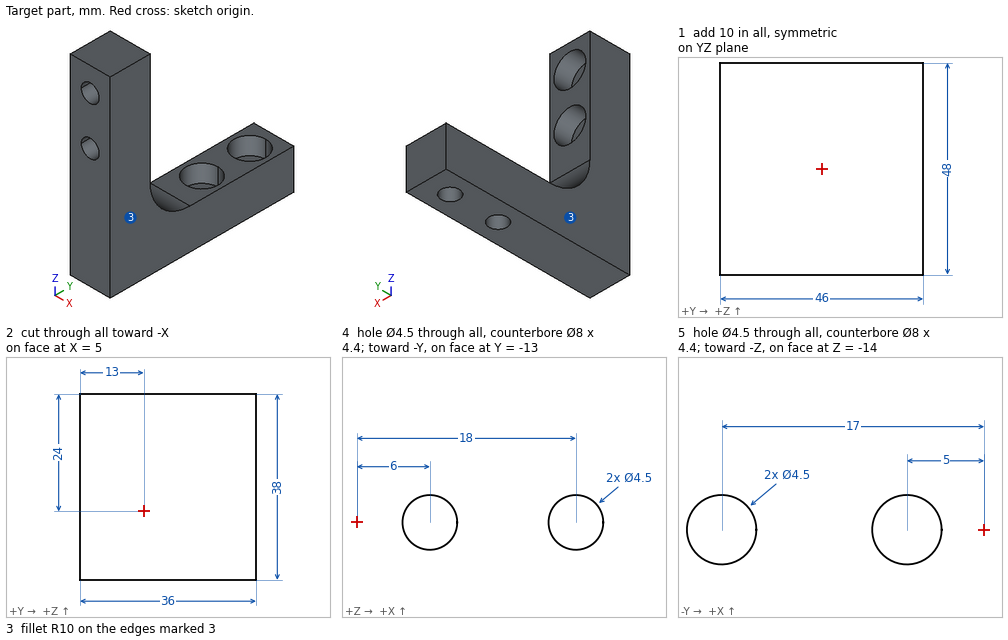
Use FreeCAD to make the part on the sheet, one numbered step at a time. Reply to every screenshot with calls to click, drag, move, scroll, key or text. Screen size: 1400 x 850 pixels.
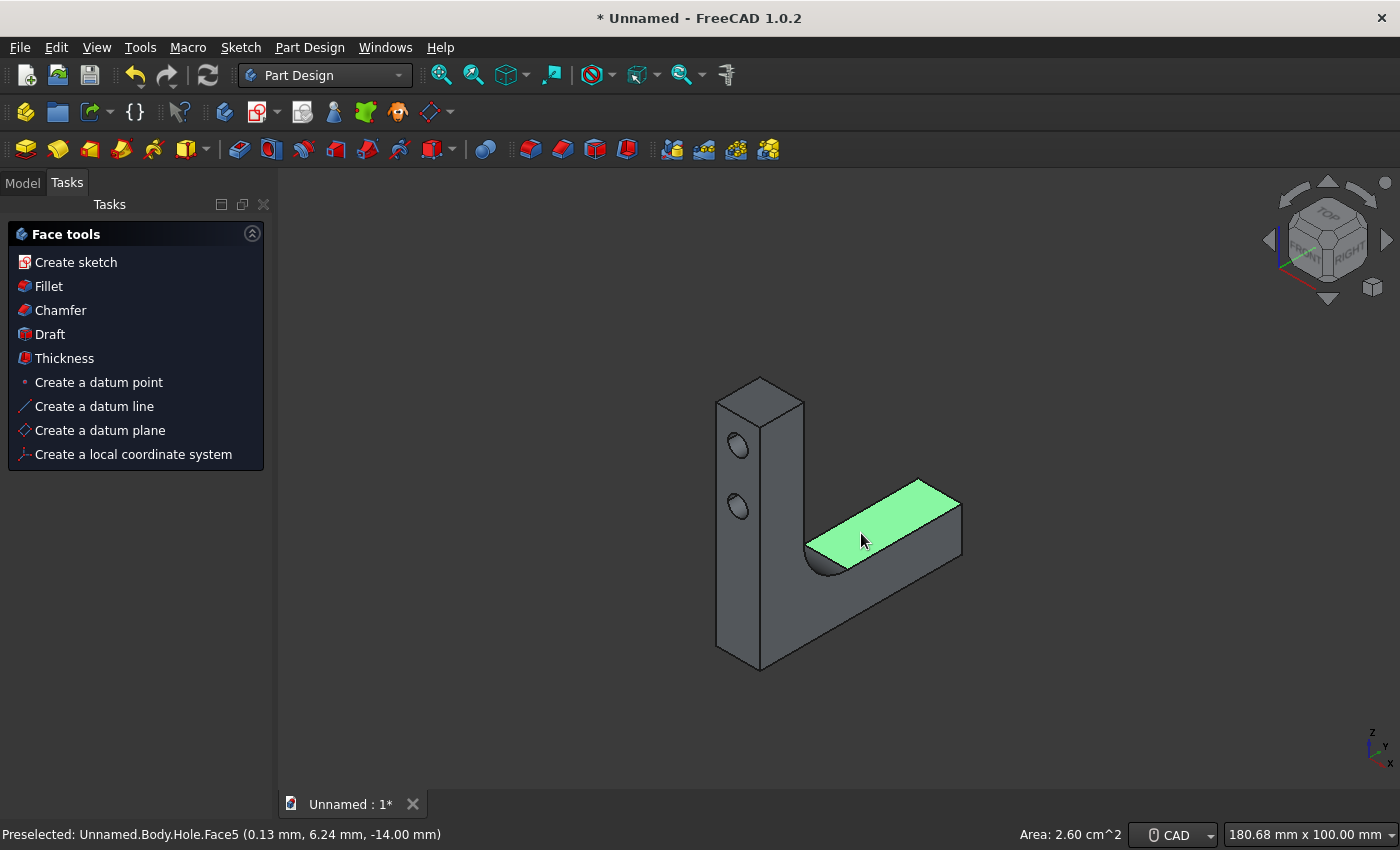
click(258, 112)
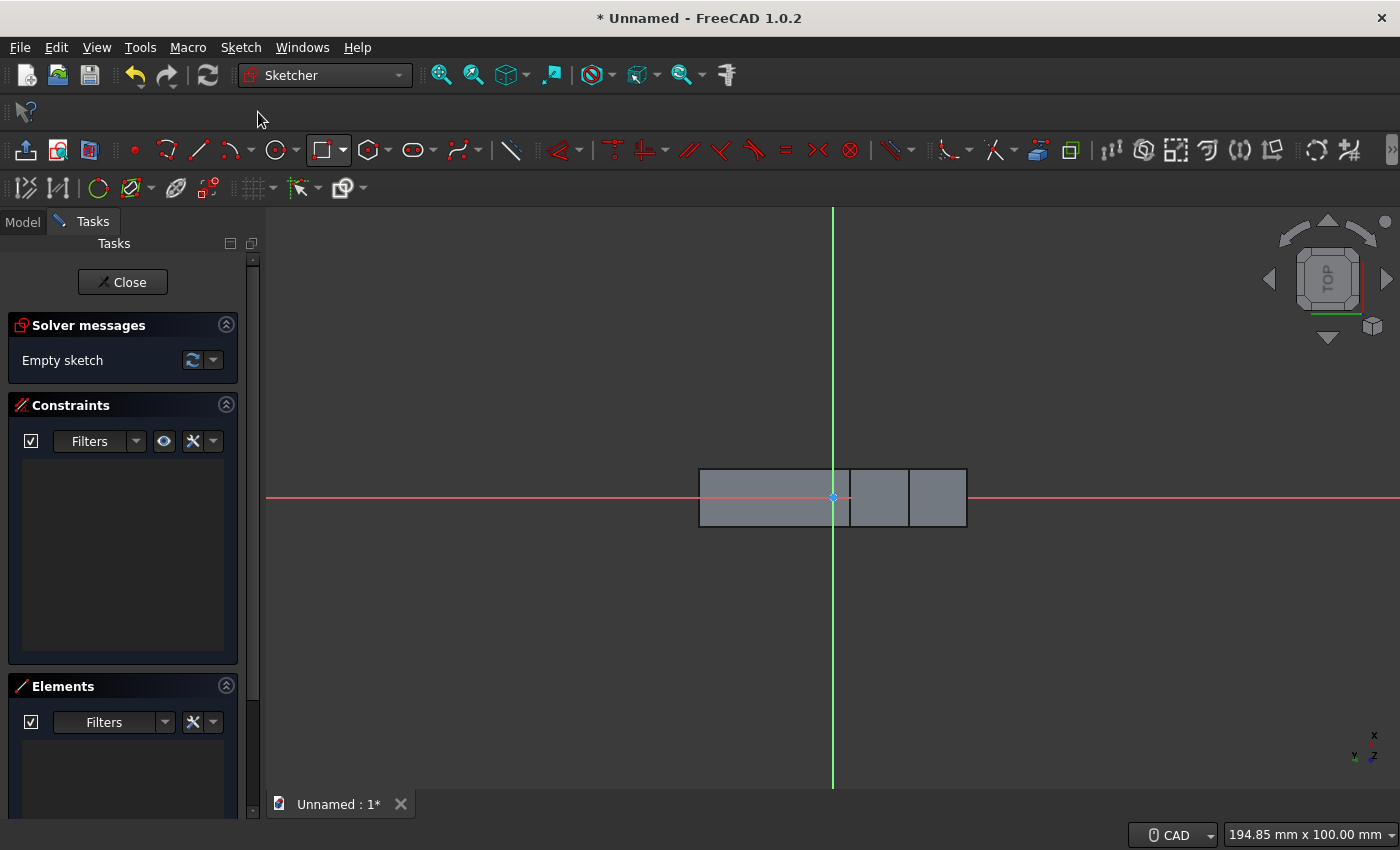
click(90, 150)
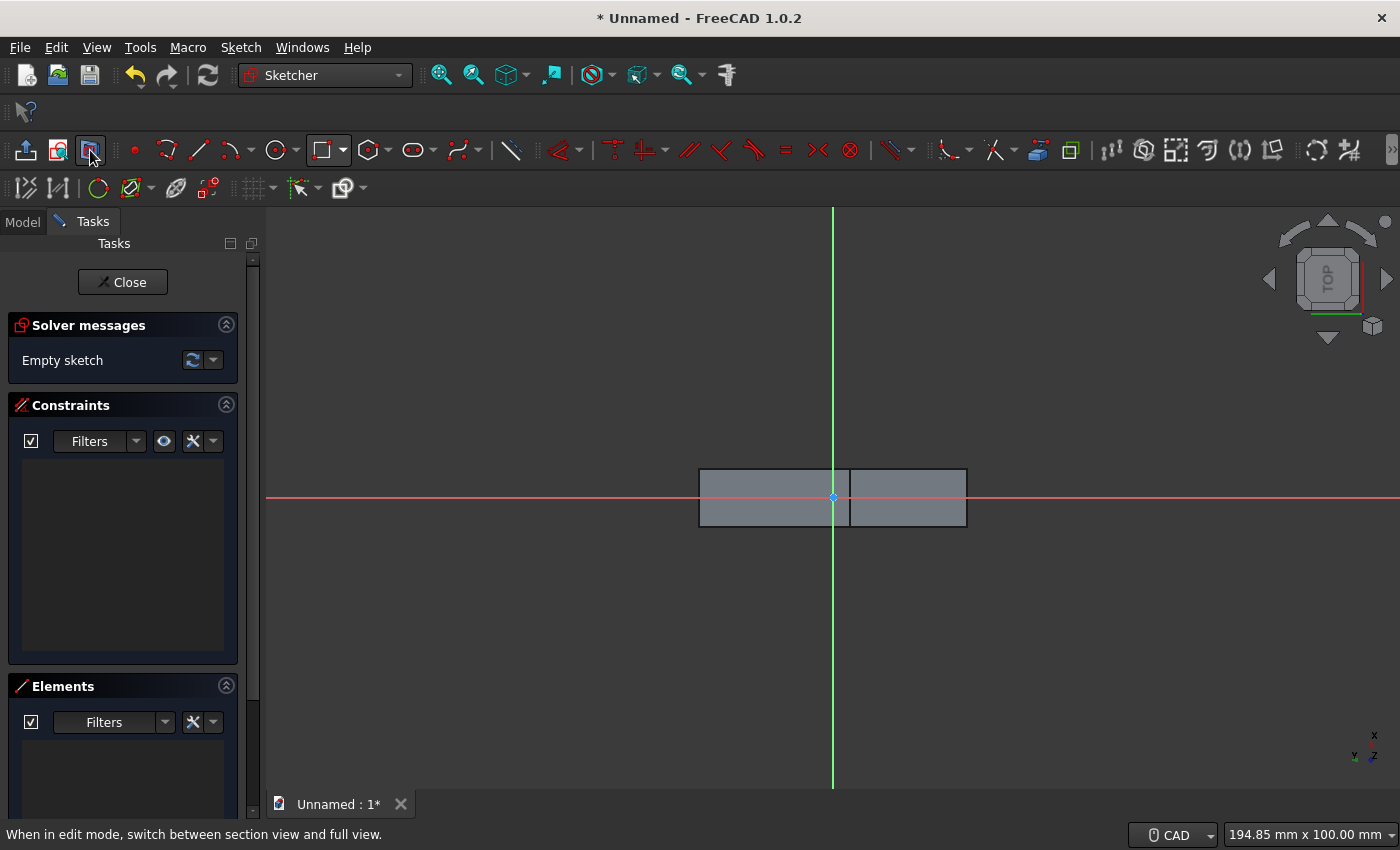
scroll(779, 498, up, 9)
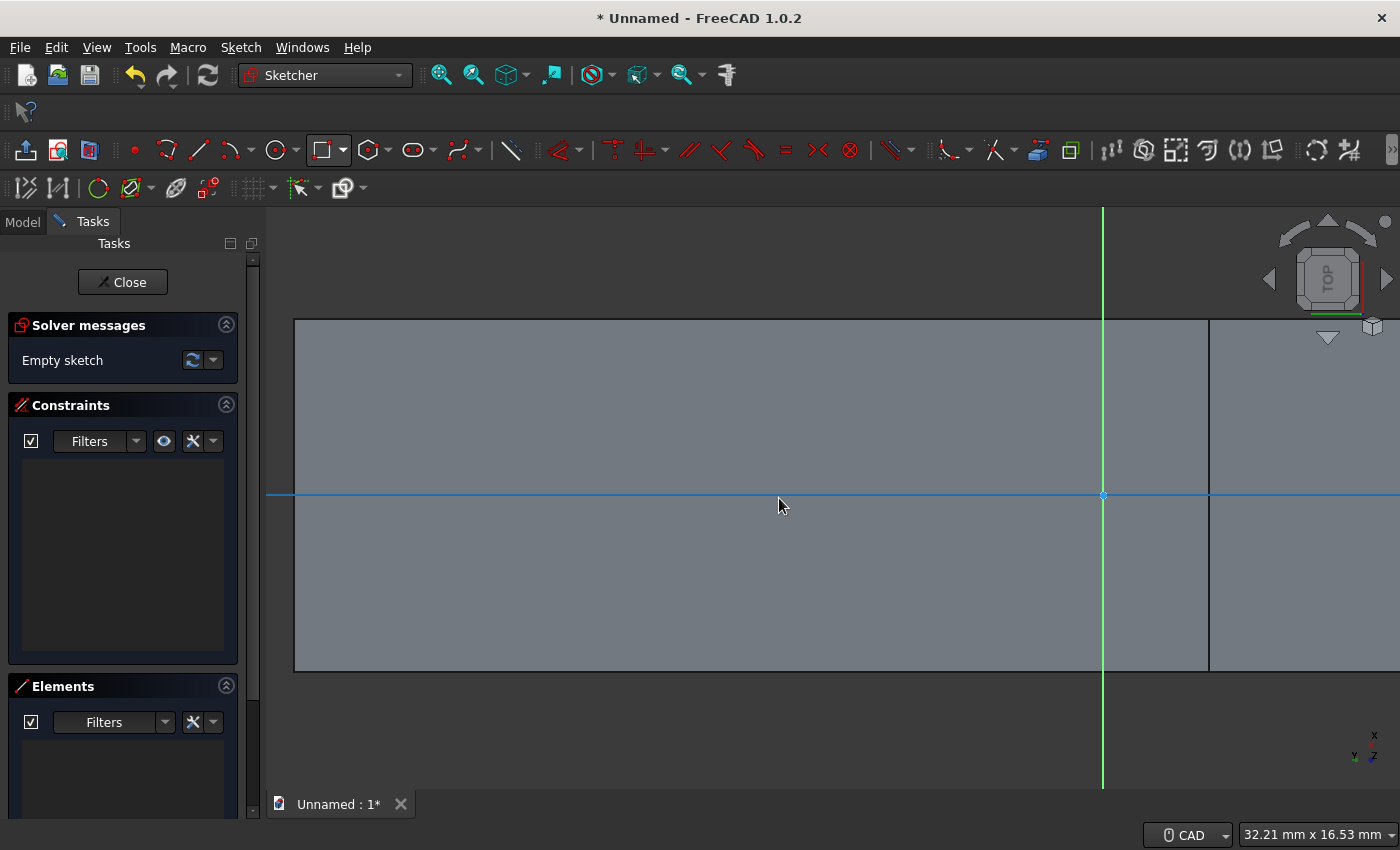
click(276, 150)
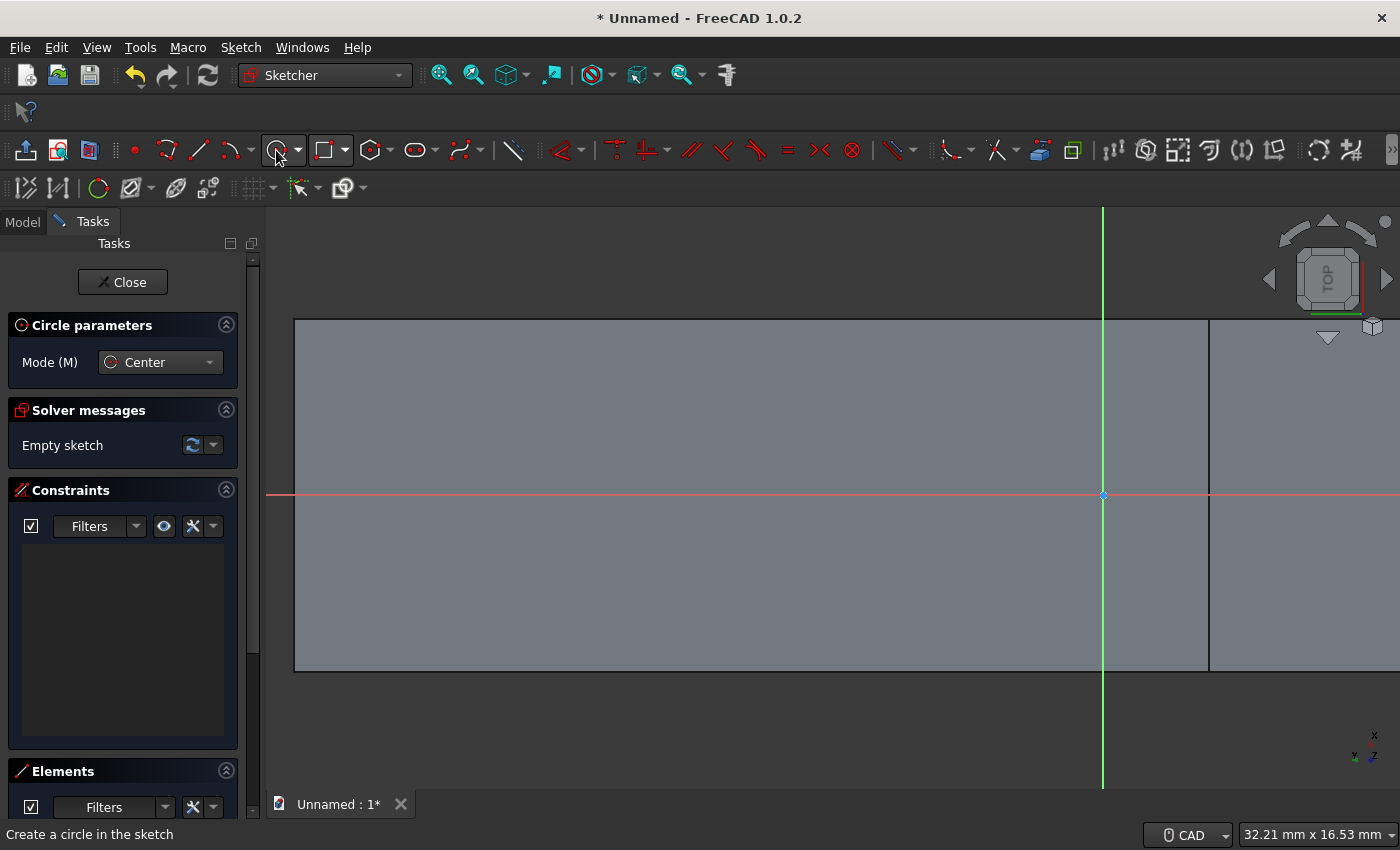
click(505, 495)
move(561, 439)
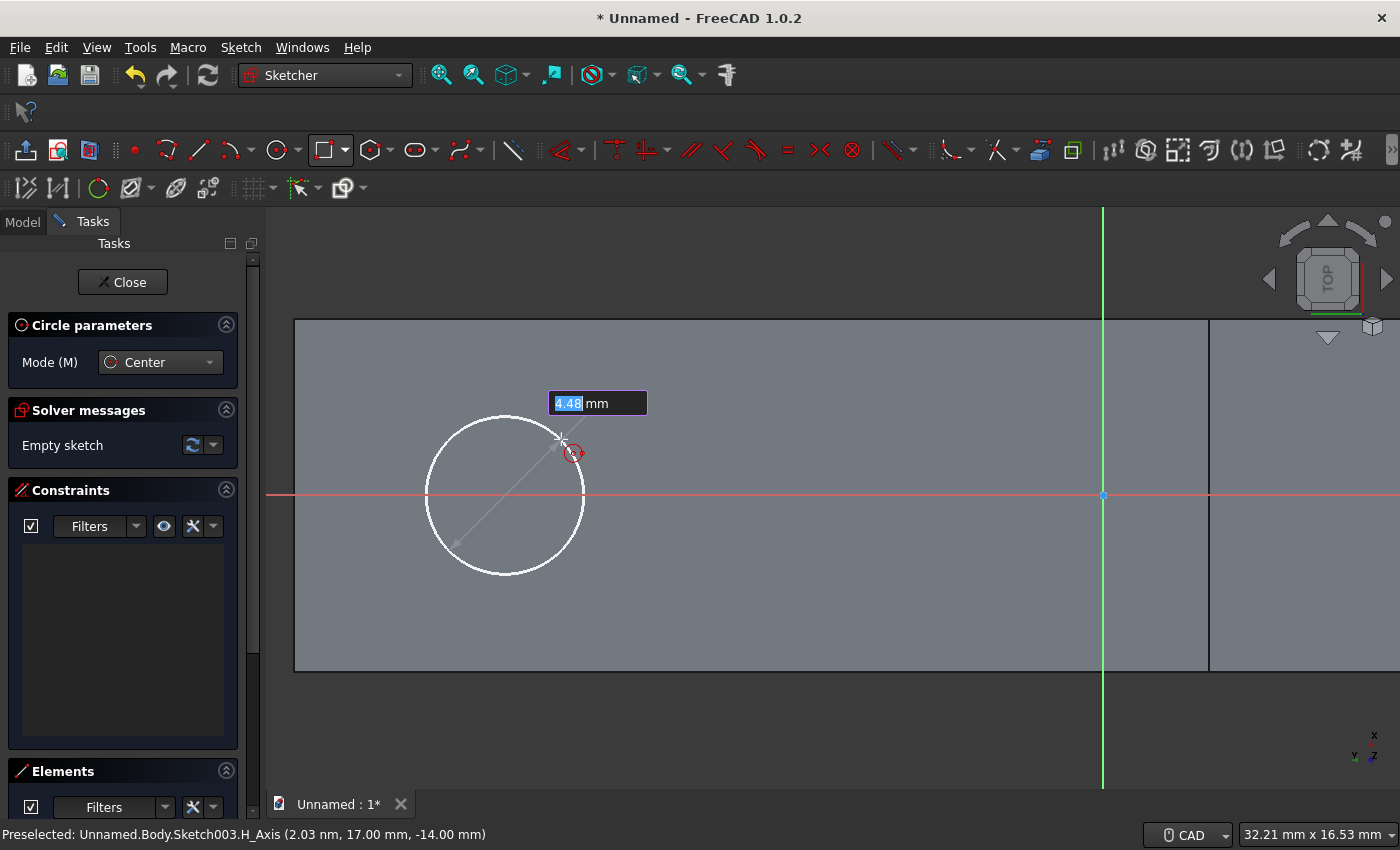
text(4.5)
key(Return)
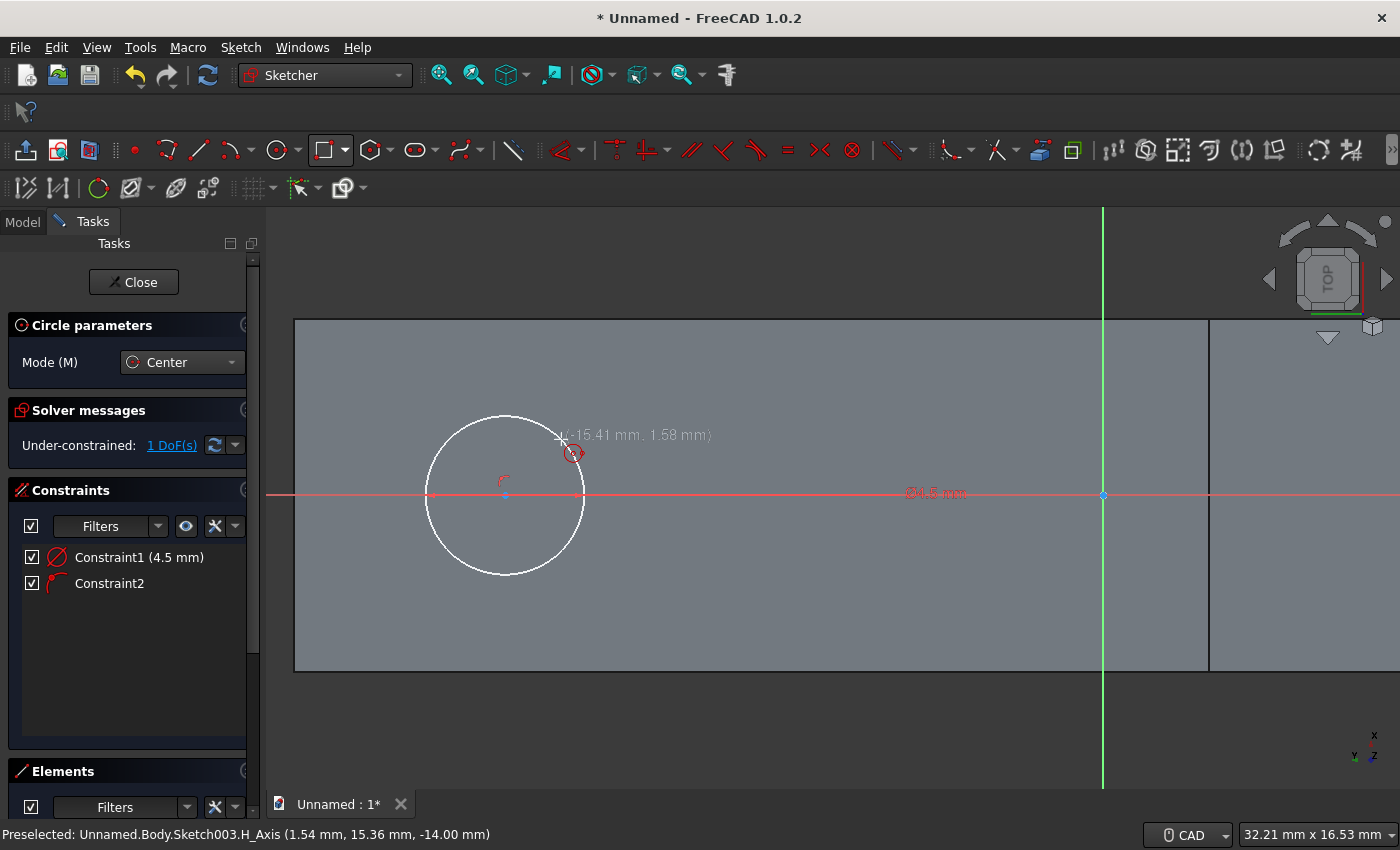
click(927, 495)
move(983, 439)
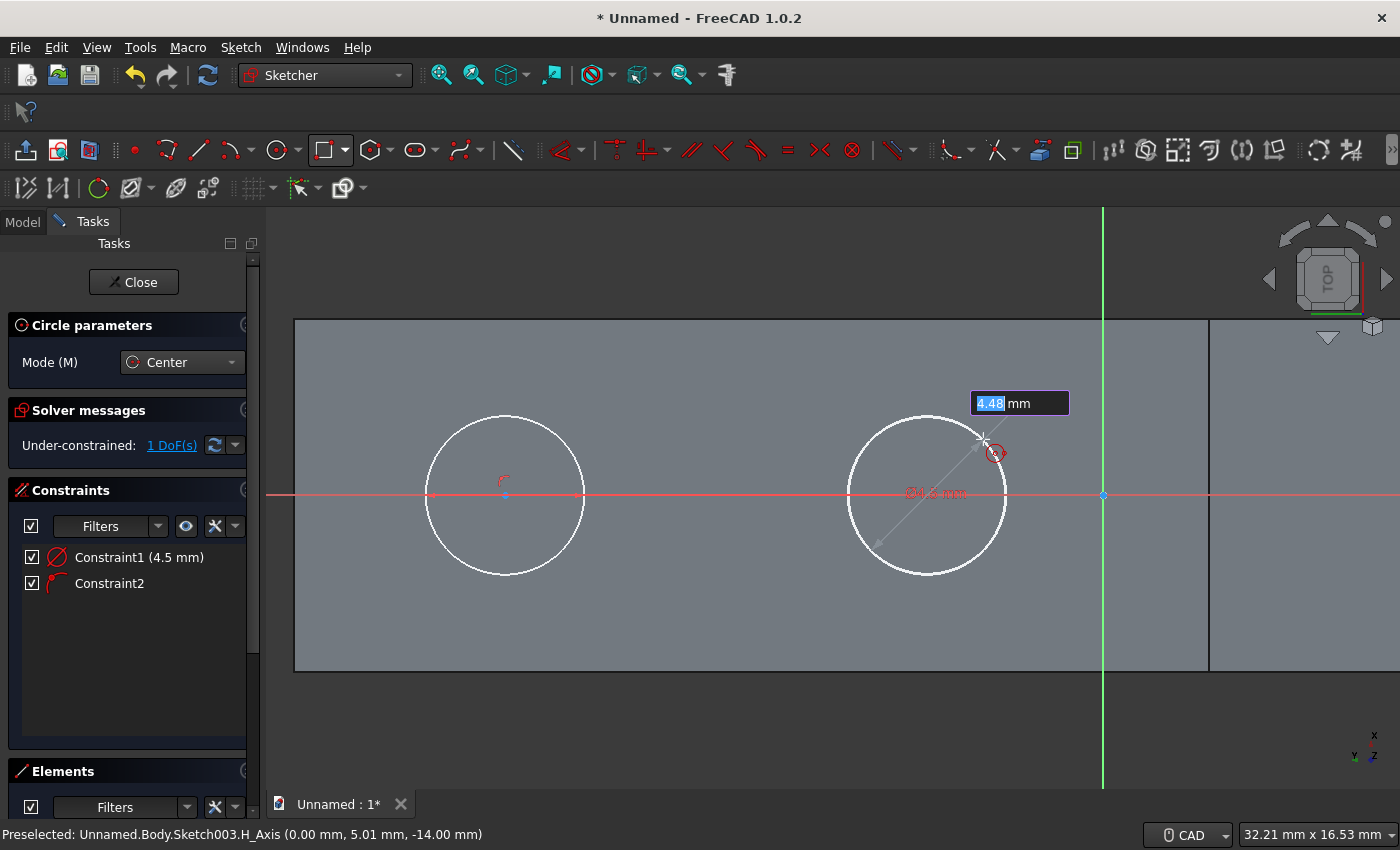
text(4.5)
key(Return)
key(Escape)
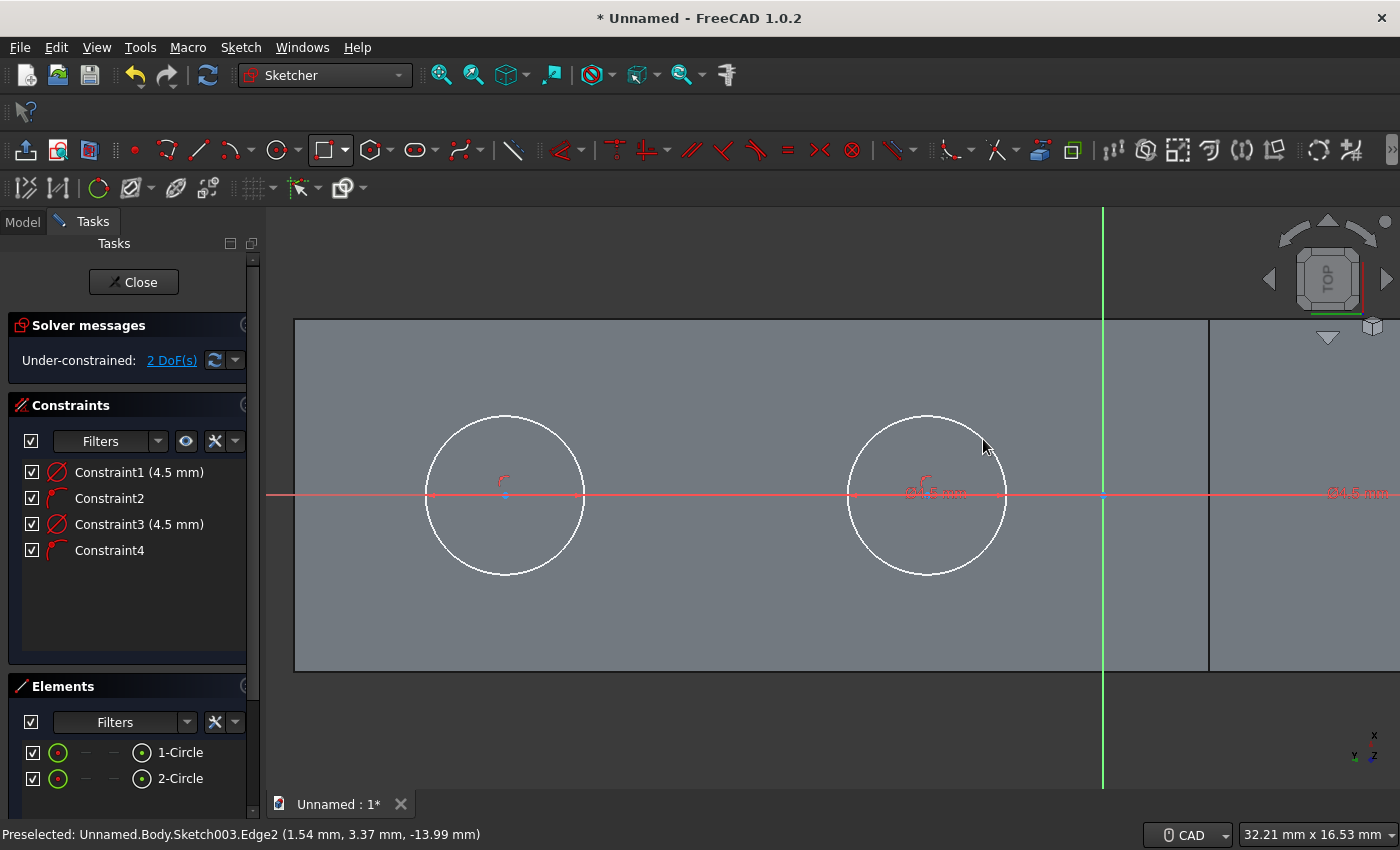
click(560, 150)